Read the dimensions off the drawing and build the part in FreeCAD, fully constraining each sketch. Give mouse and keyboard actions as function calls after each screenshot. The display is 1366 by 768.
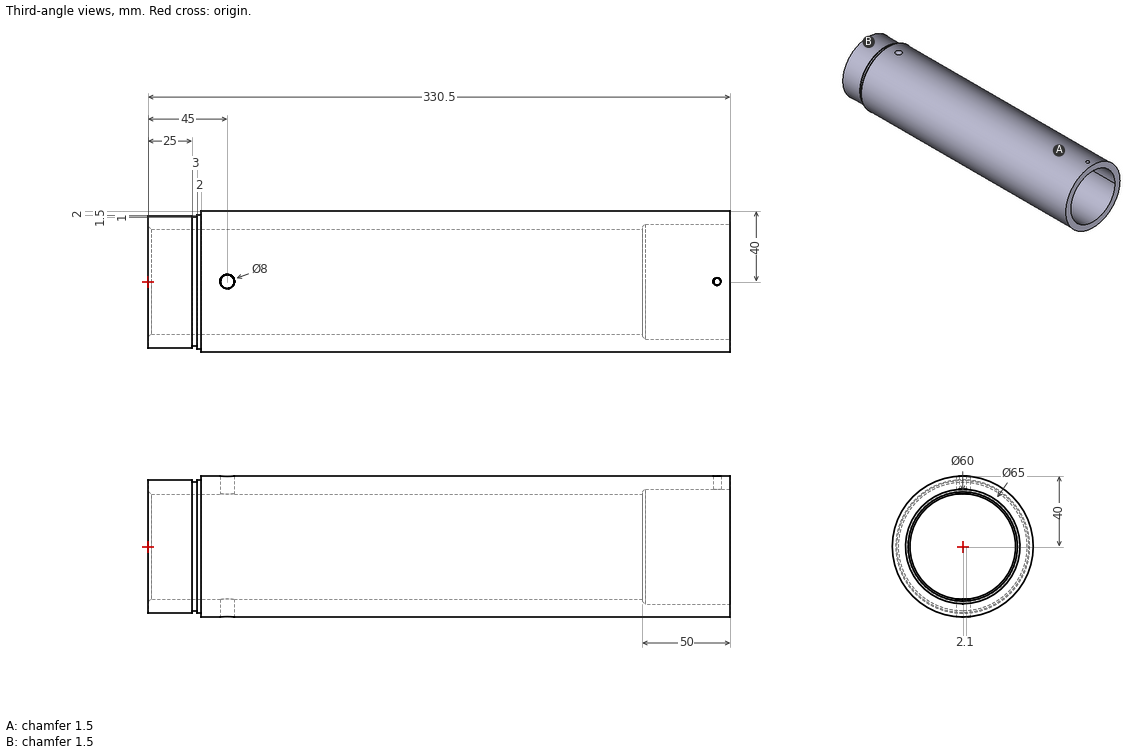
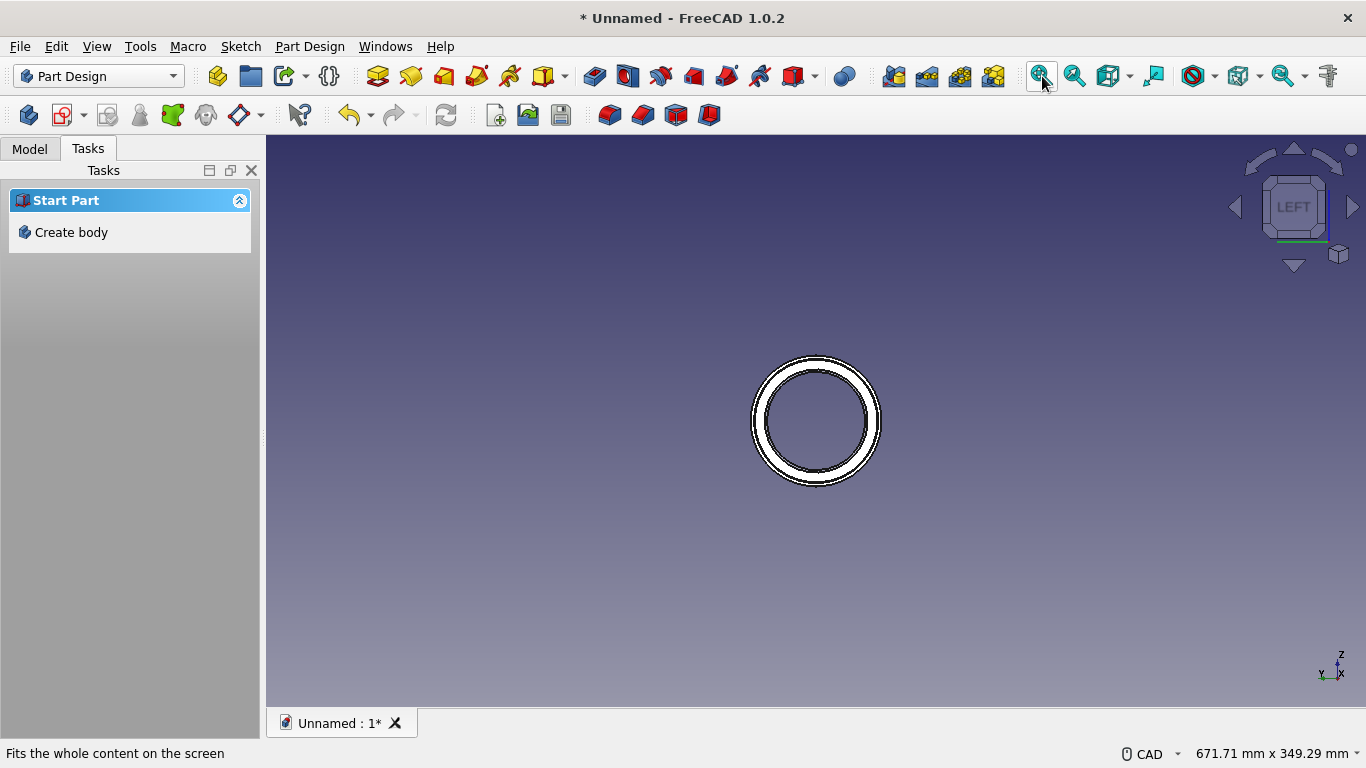
click(30, 148)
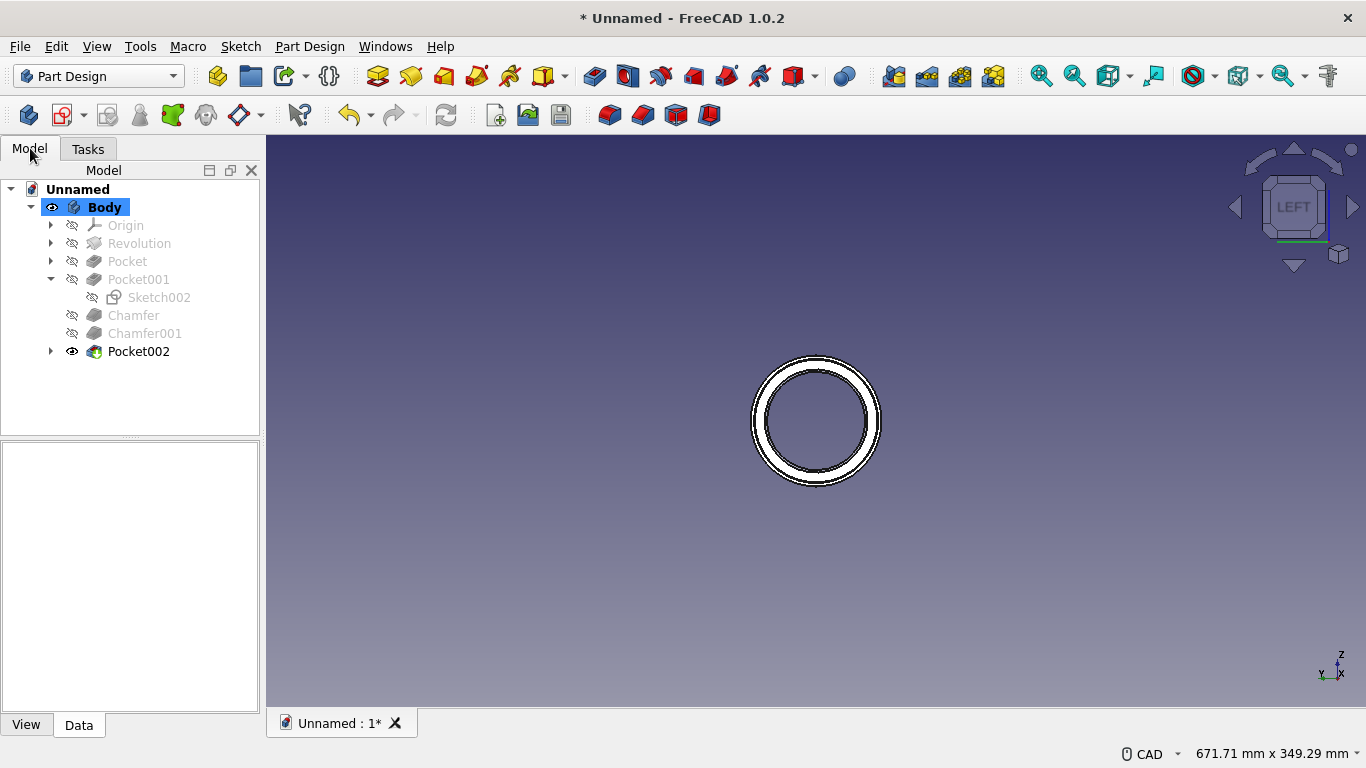
click(51, 225)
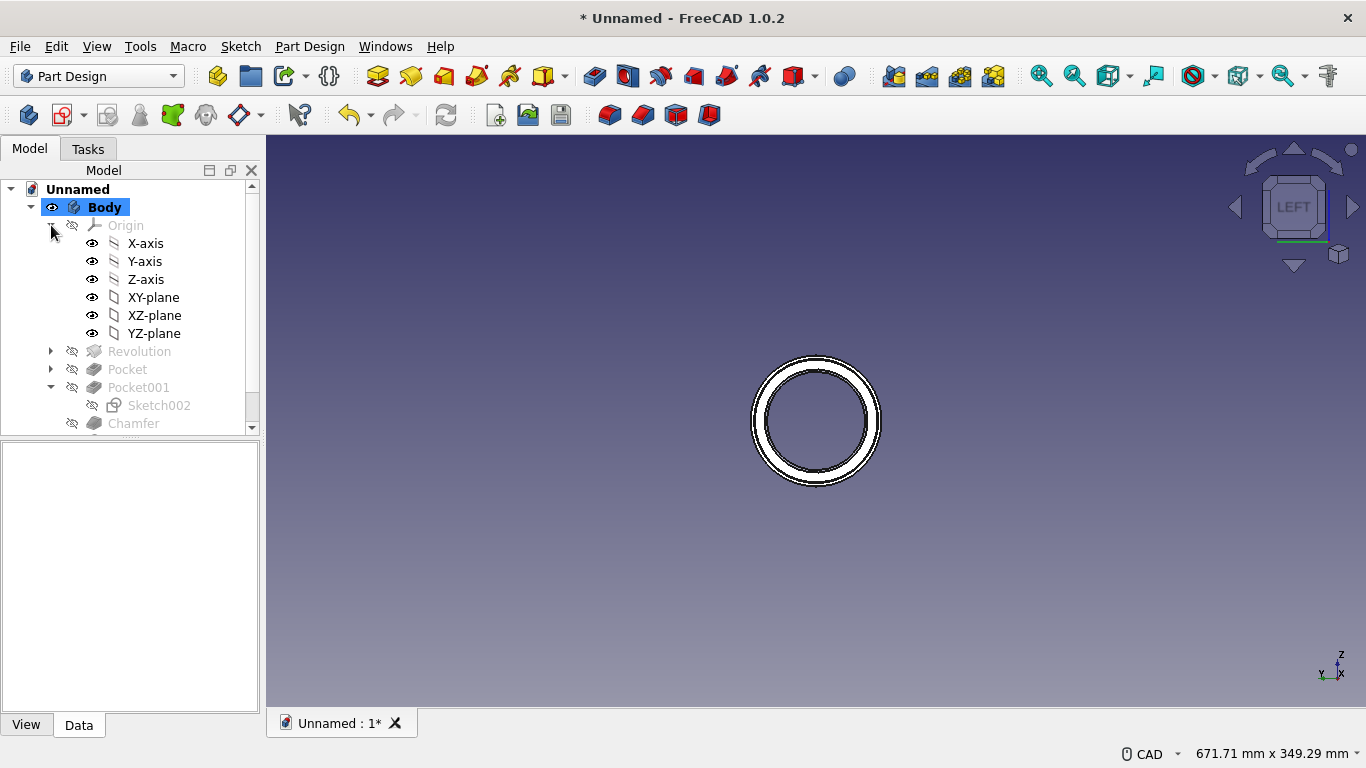
click(137, 333)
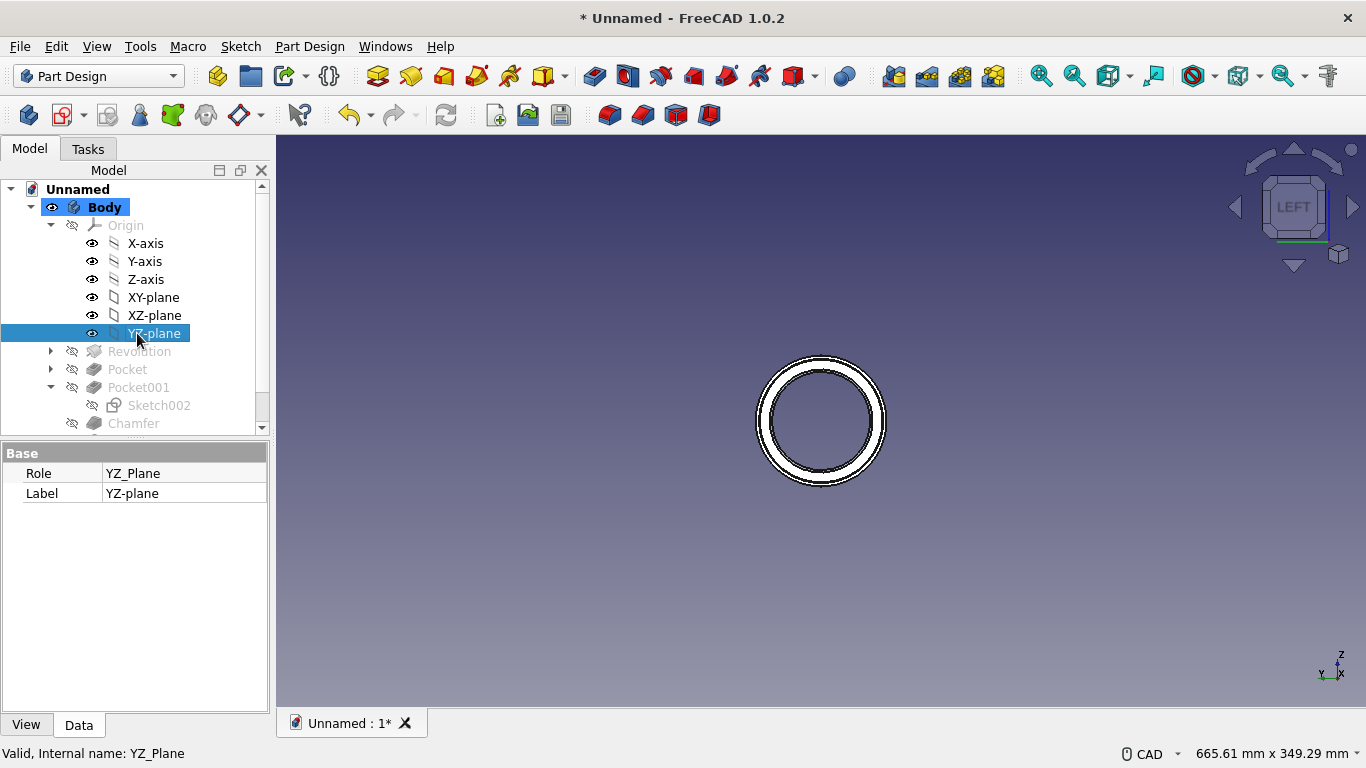
click(238, 116)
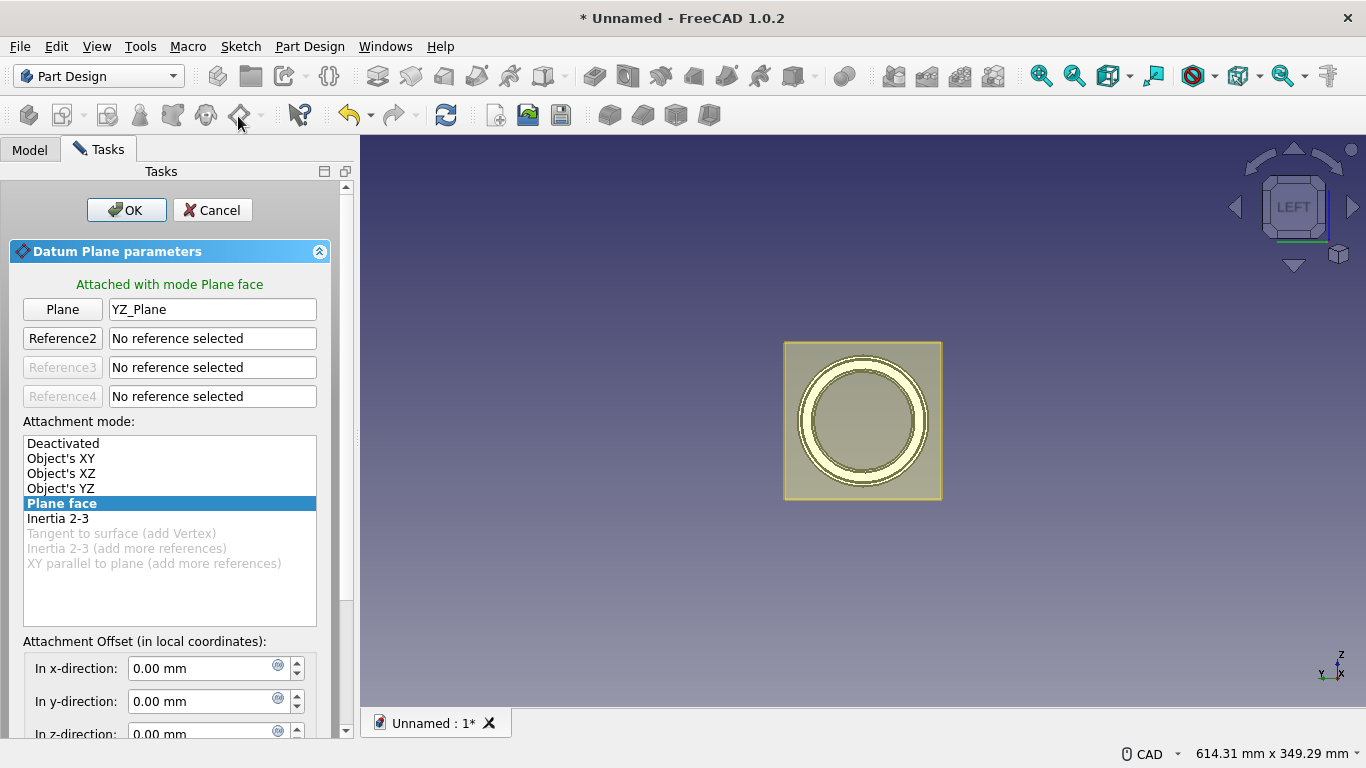
scroll(346, 460, down, 2)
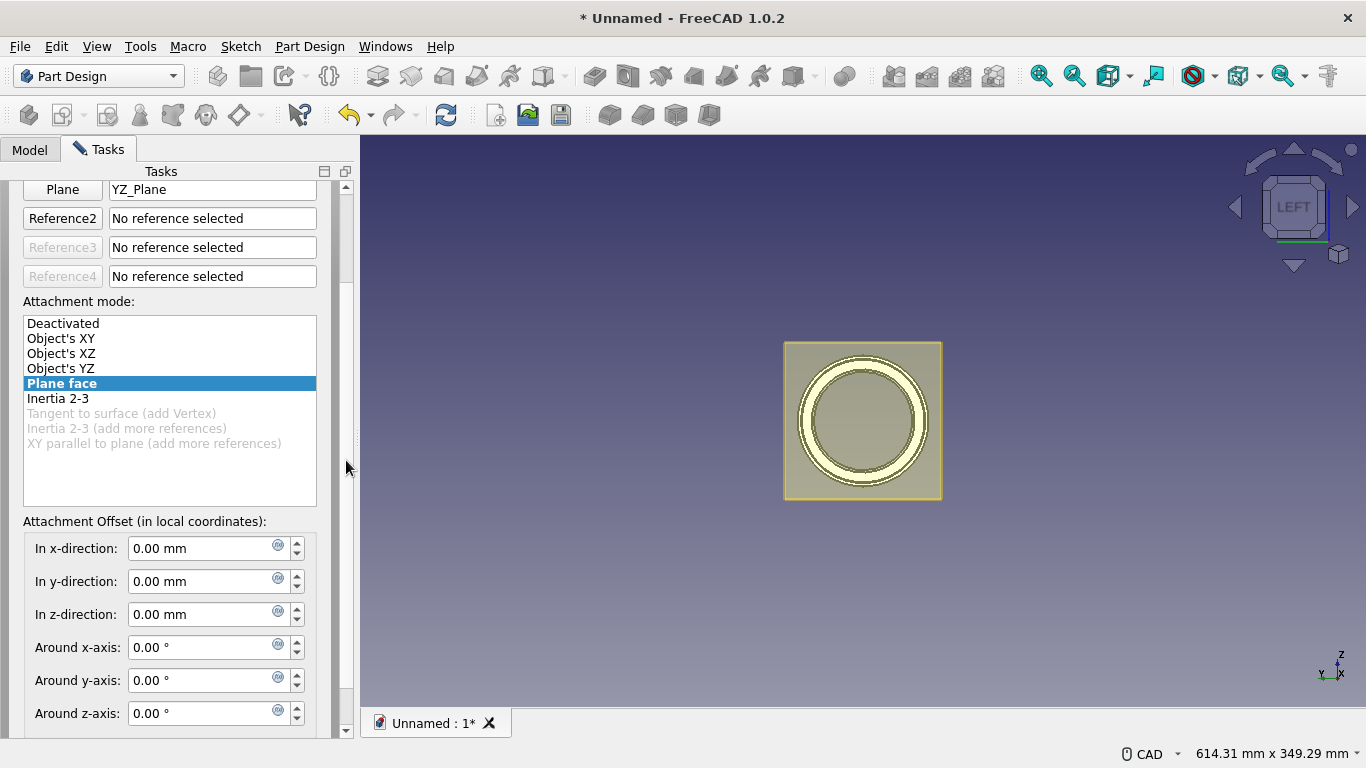
triple_click(210, 614)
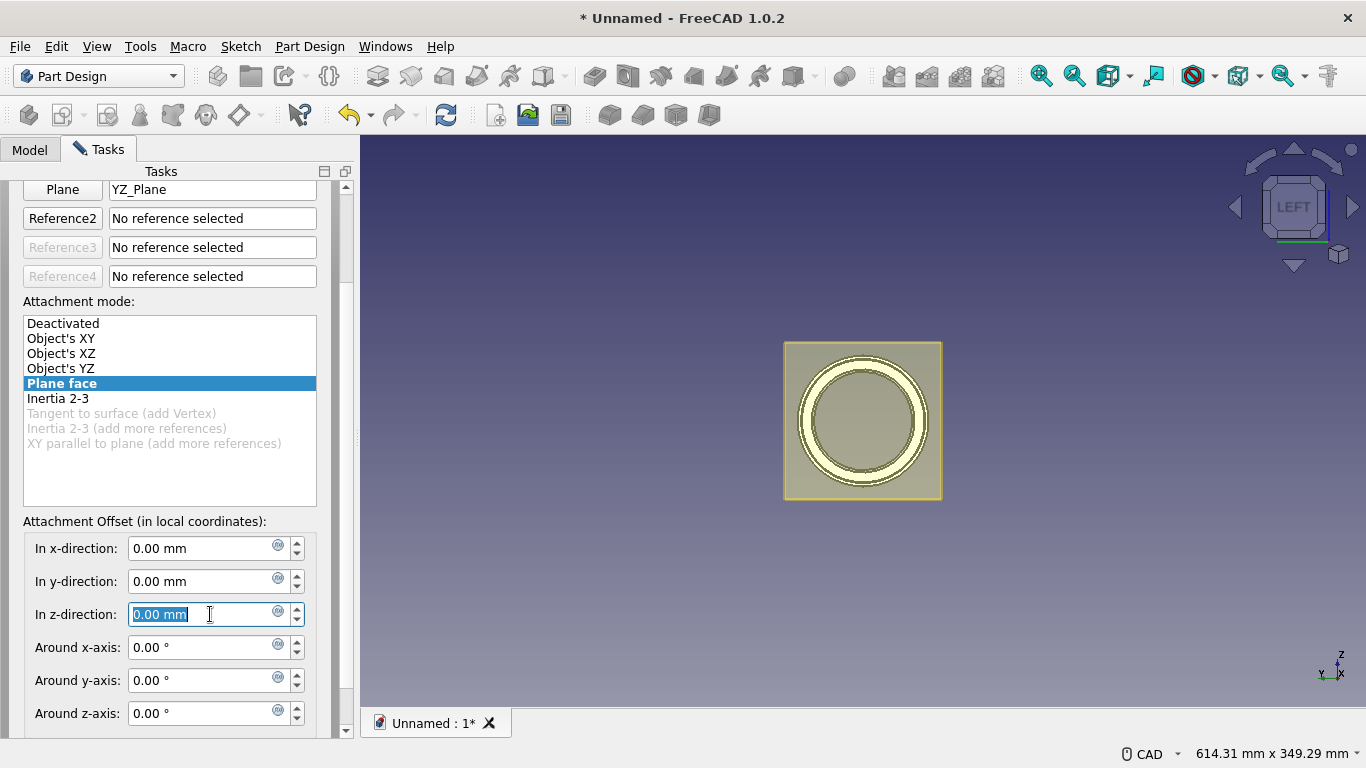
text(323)
key(Tab)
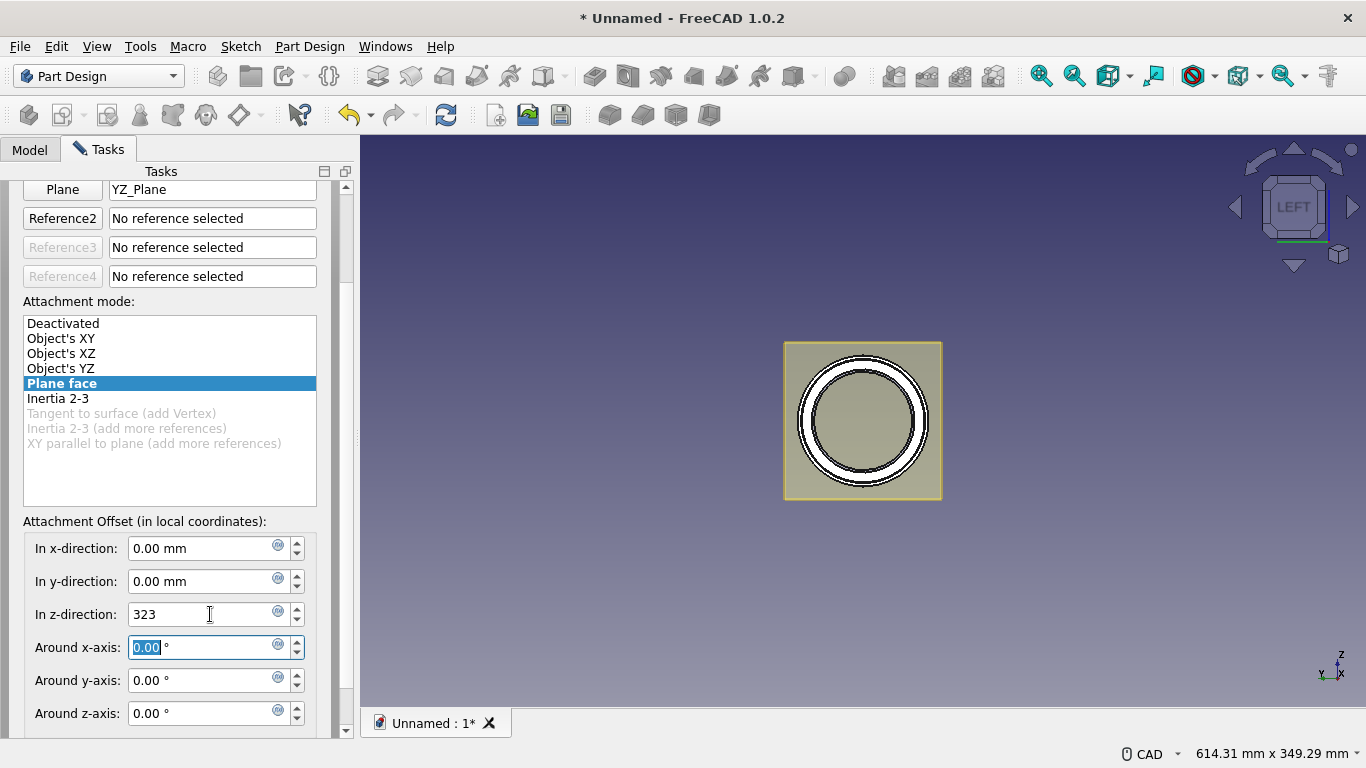
scroll(346, 460, up, 3)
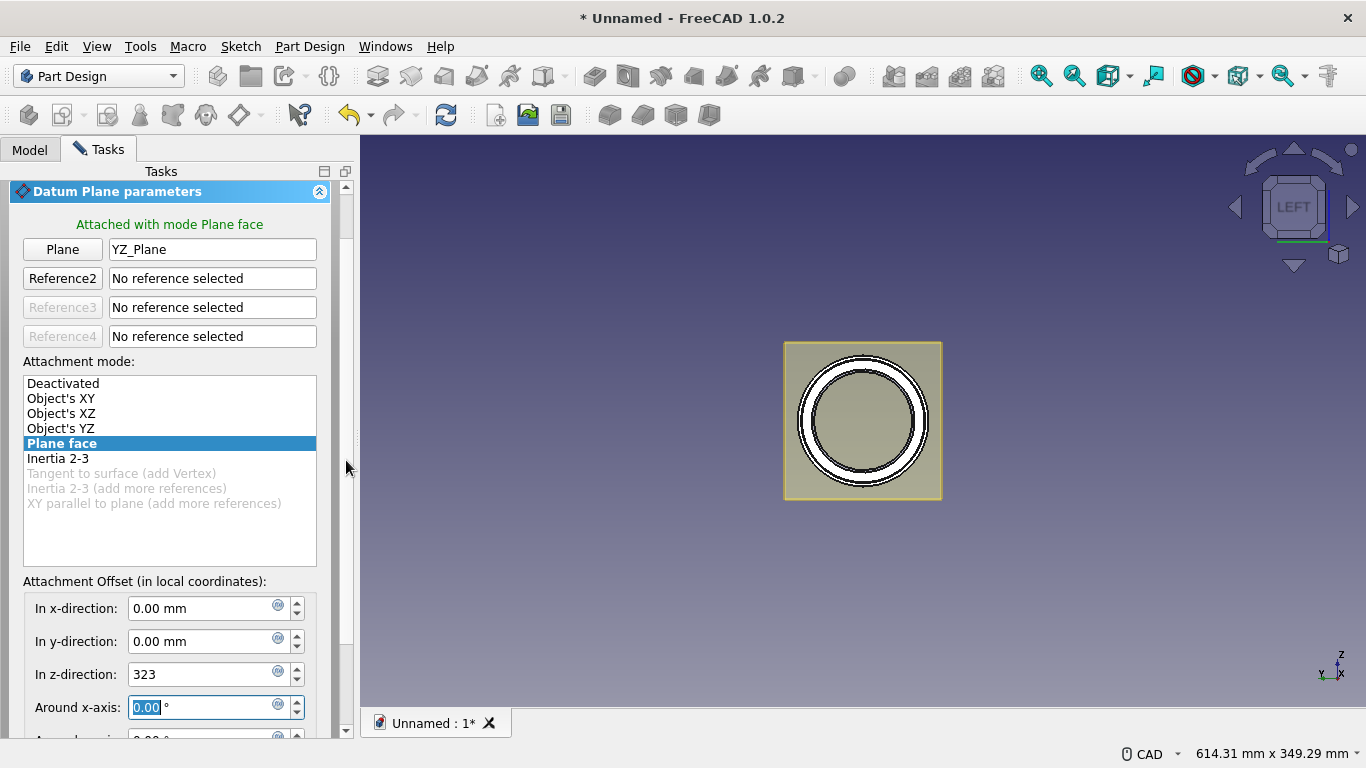
click(127, 210)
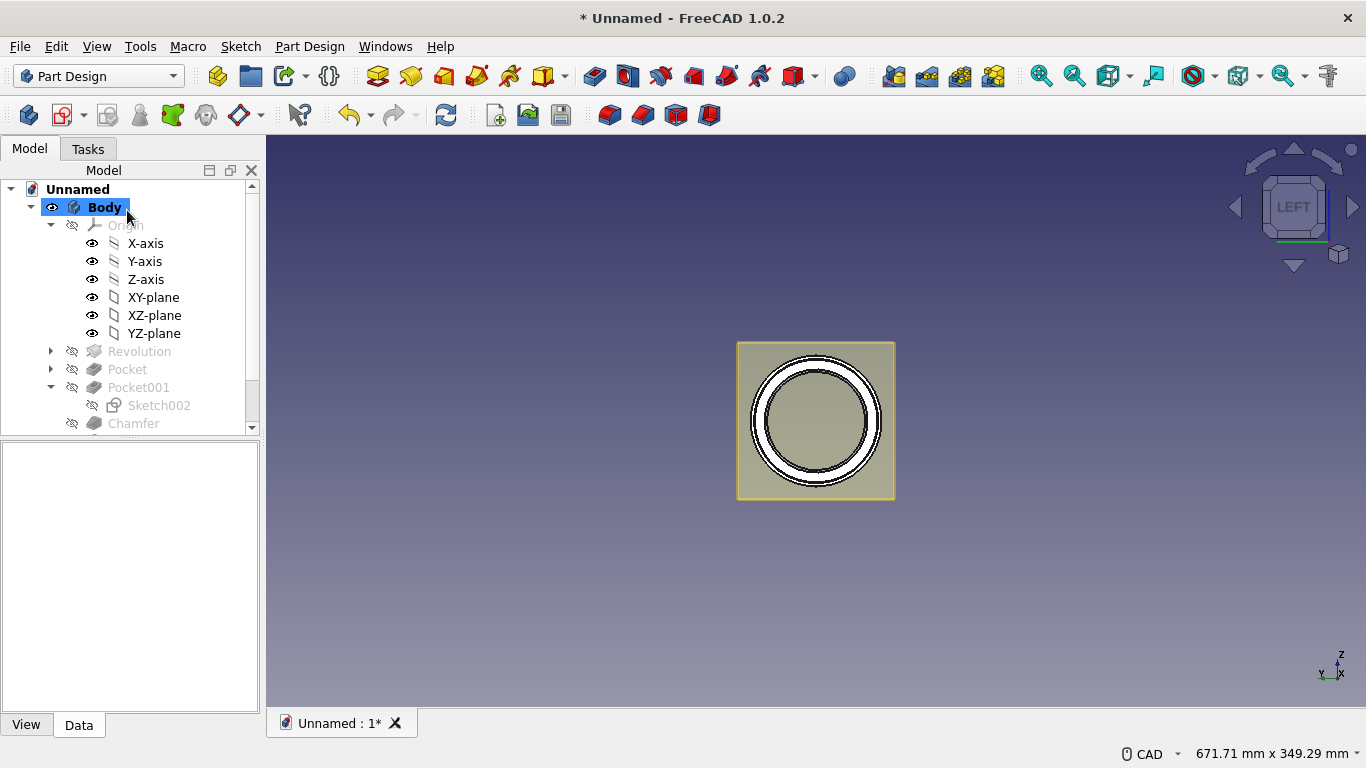
scroll(101, 311, down, 3)